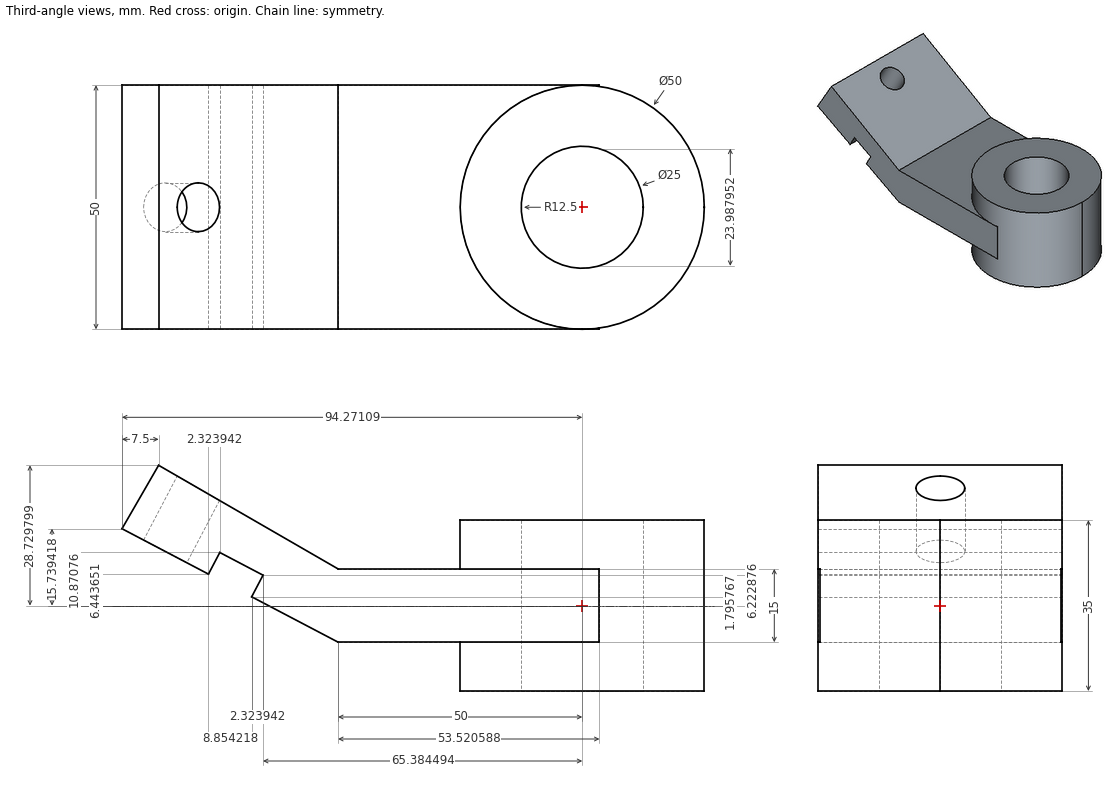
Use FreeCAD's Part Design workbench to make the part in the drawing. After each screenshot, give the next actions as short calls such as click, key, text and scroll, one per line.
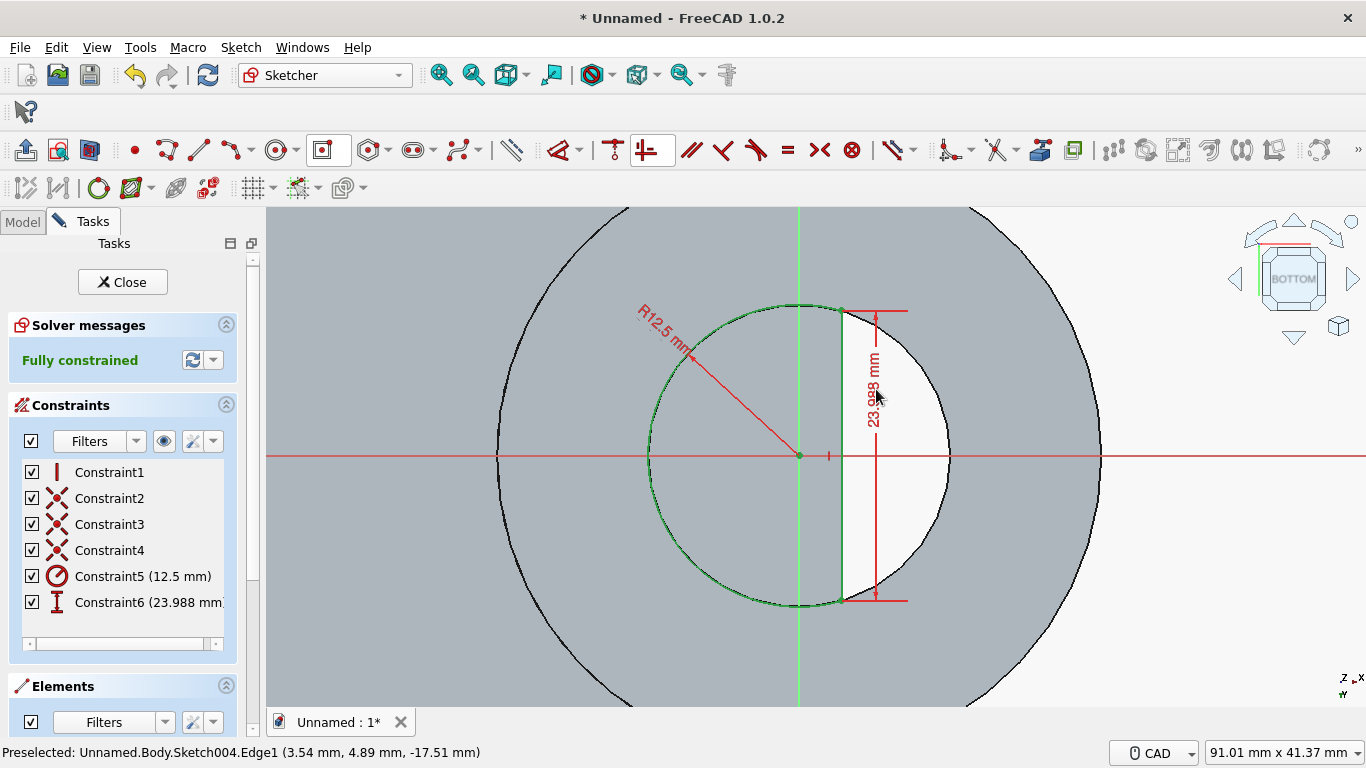
click(123, 282)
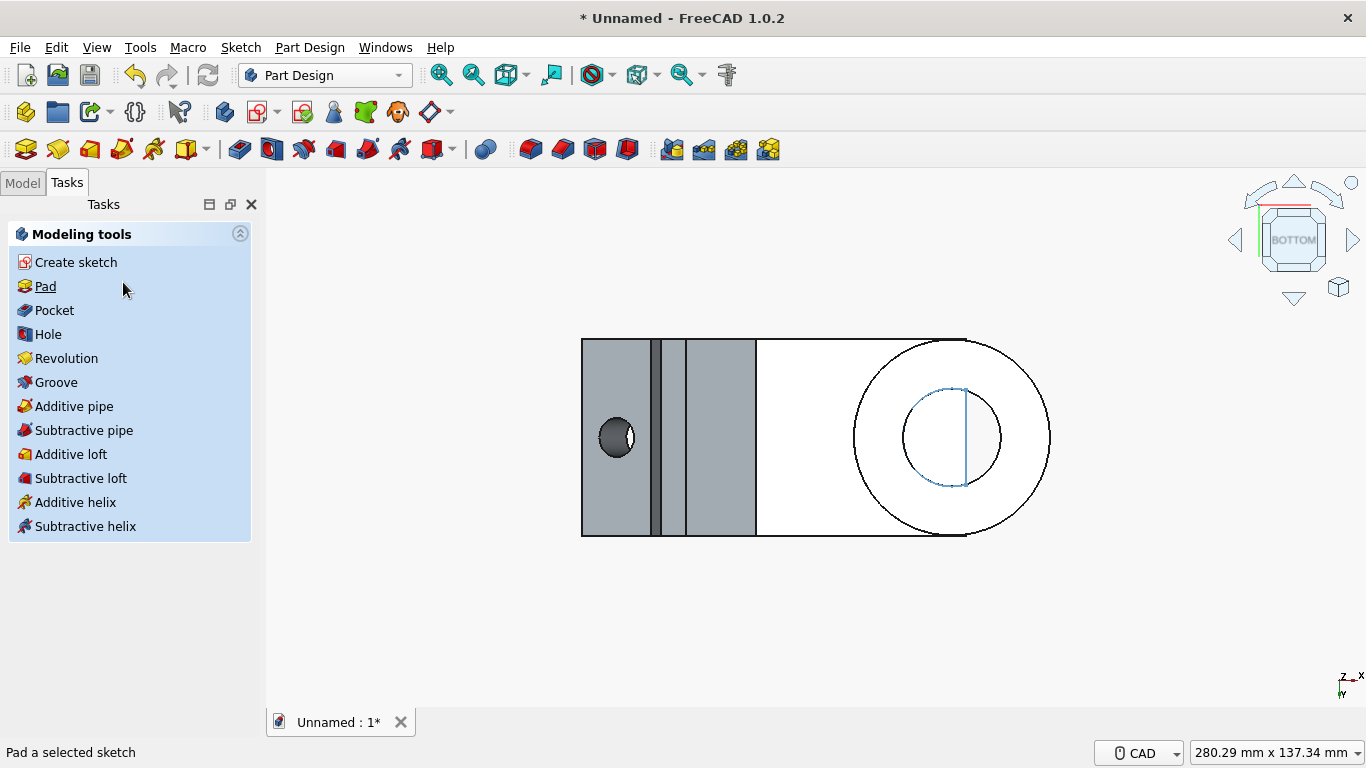
click(240, 150)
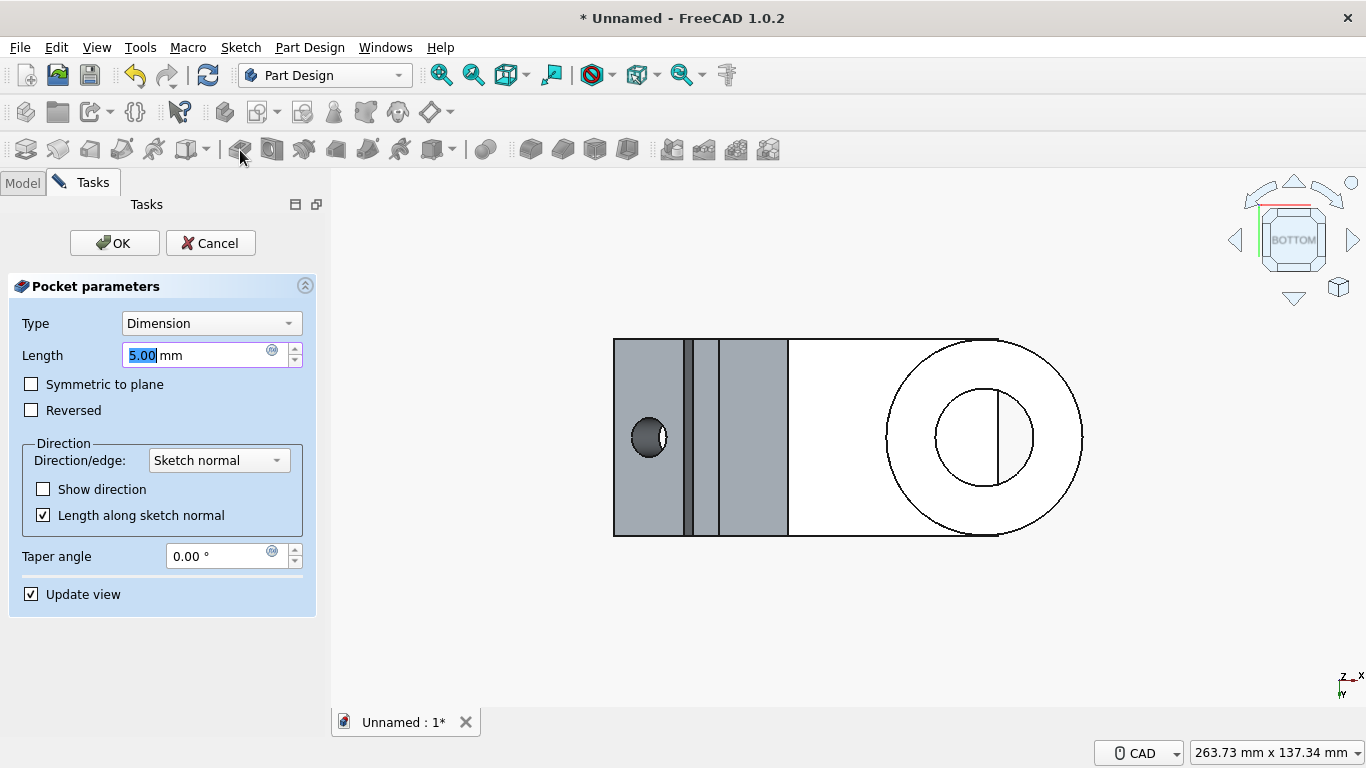
click(212, 324)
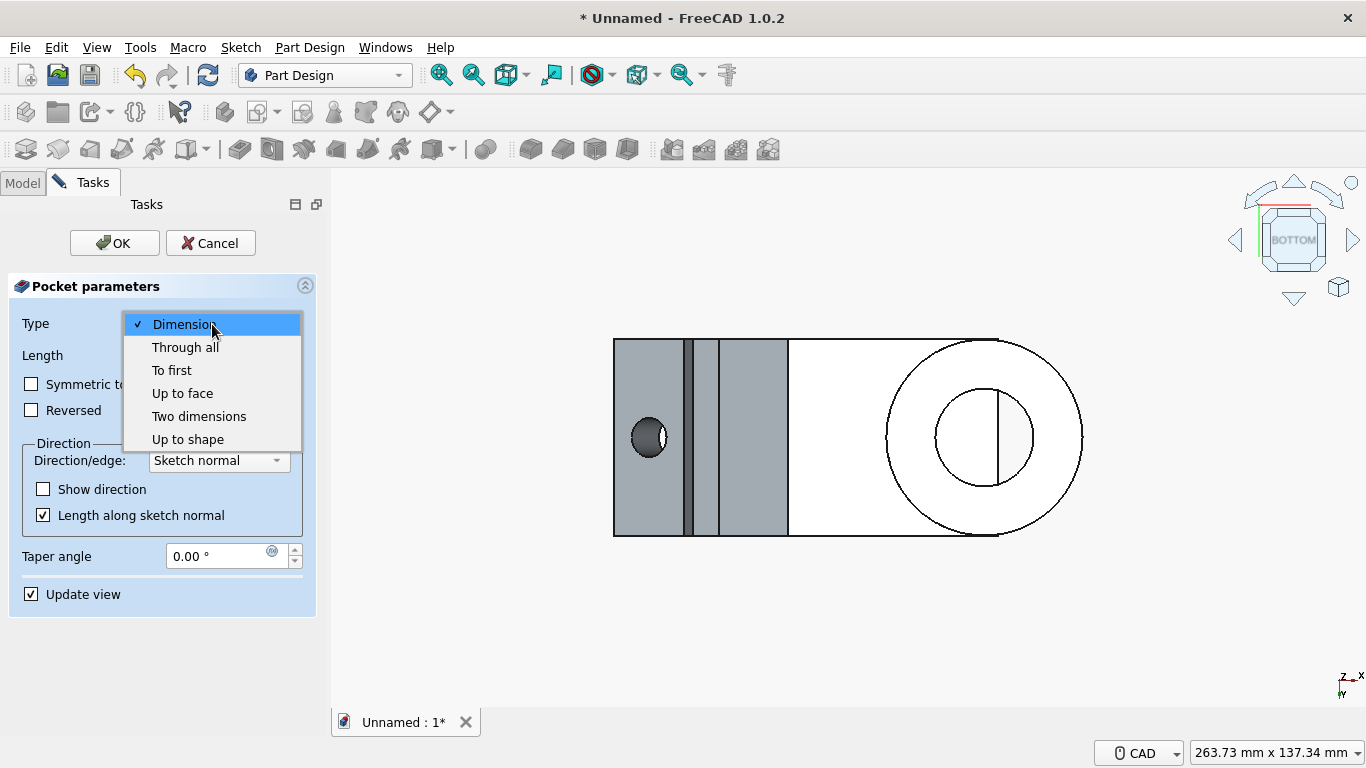
click(212, 348)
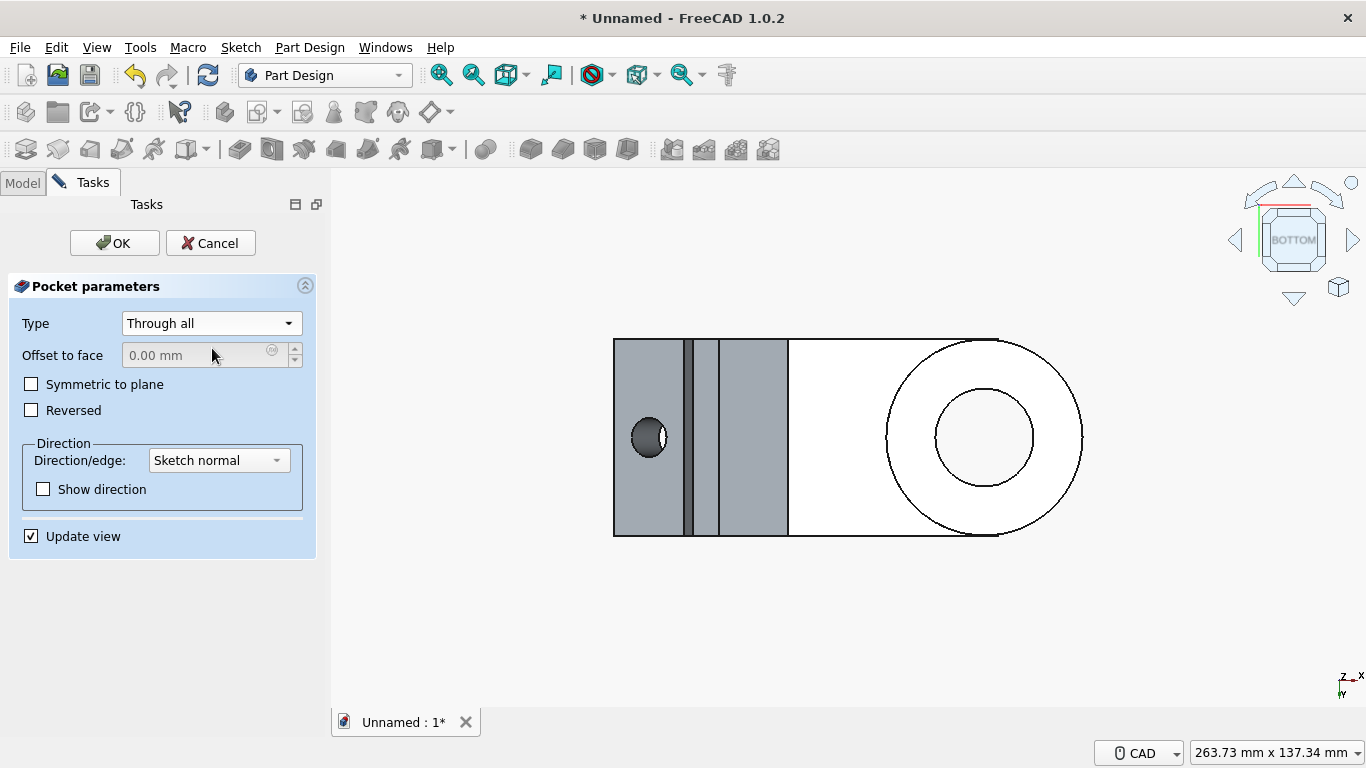
click(115, 243)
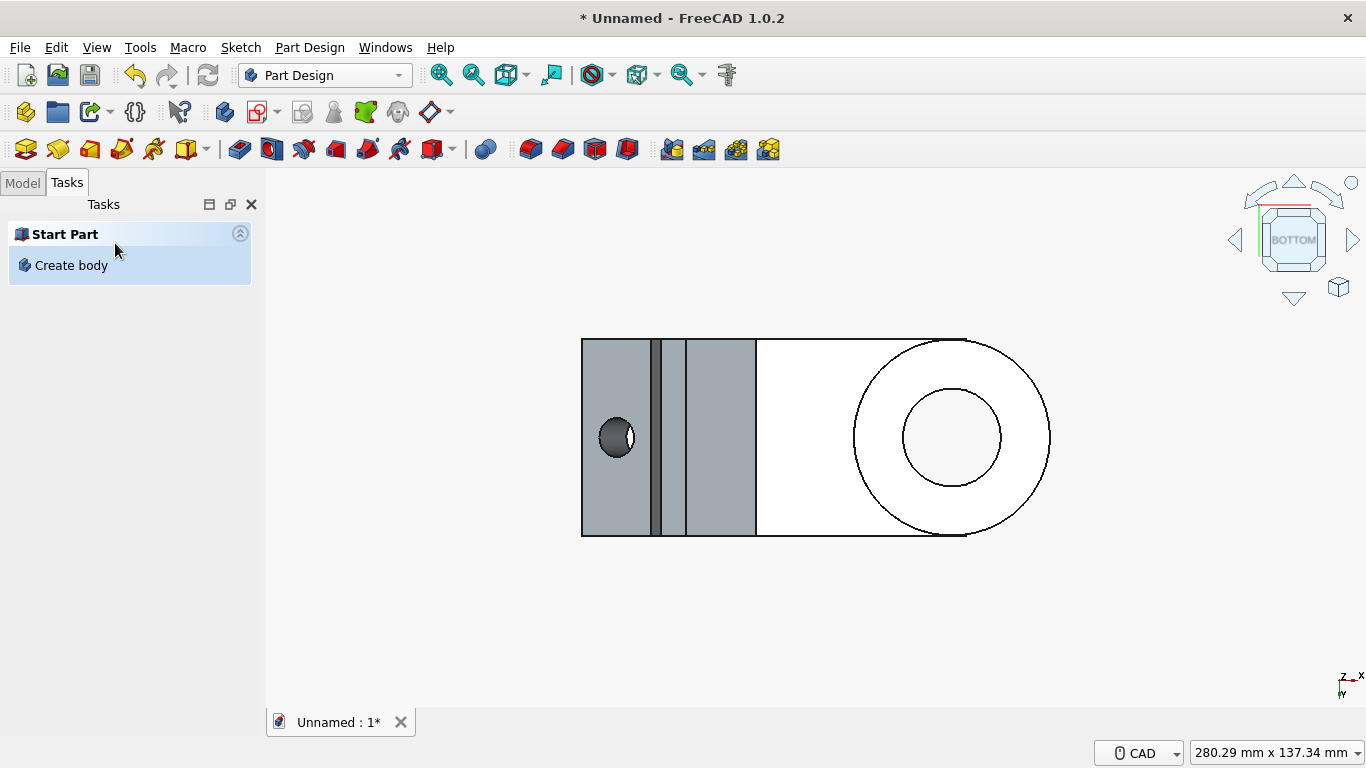
key(0)